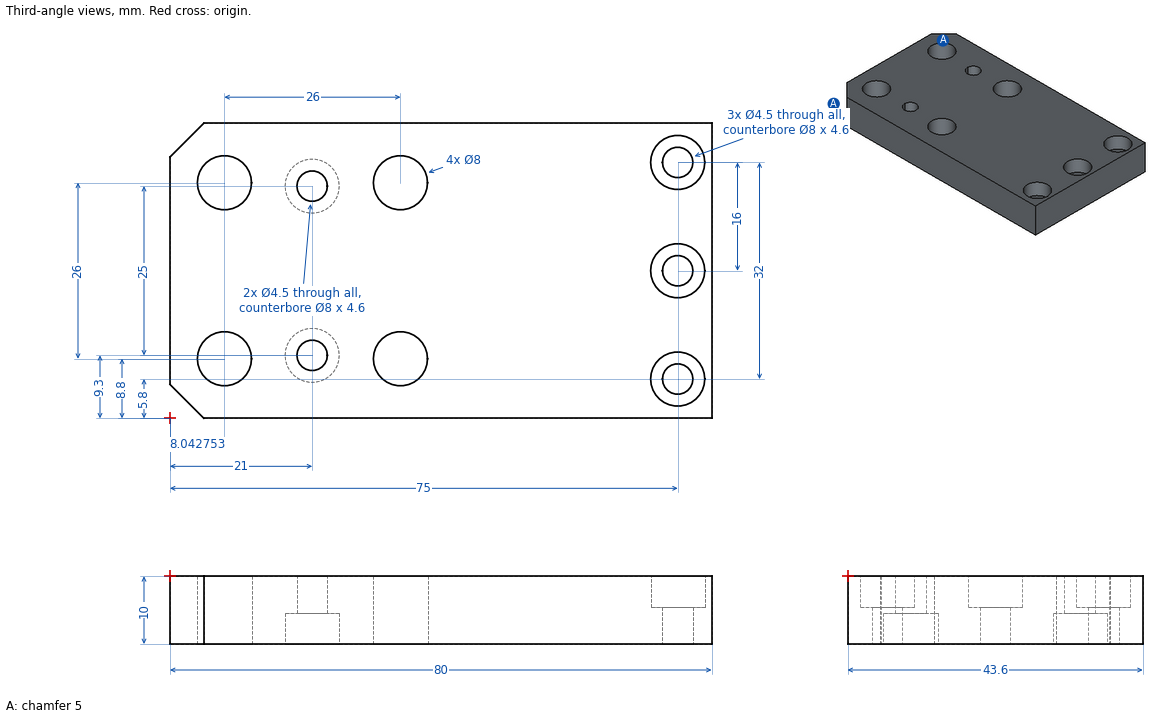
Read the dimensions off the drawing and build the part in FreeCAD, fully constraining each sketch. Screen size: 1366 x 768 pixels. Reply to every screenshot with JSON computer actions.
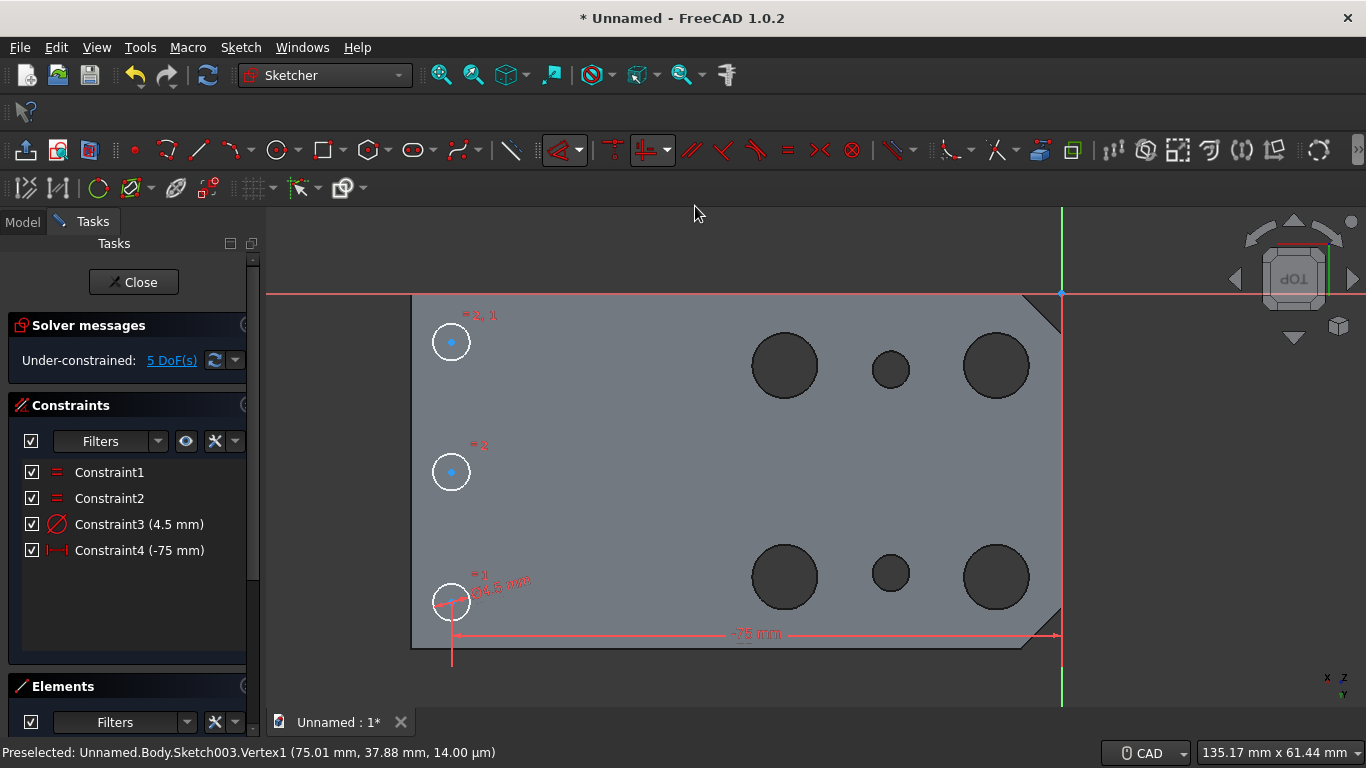
{"action": "left_click", "coordinate": [451, 342]}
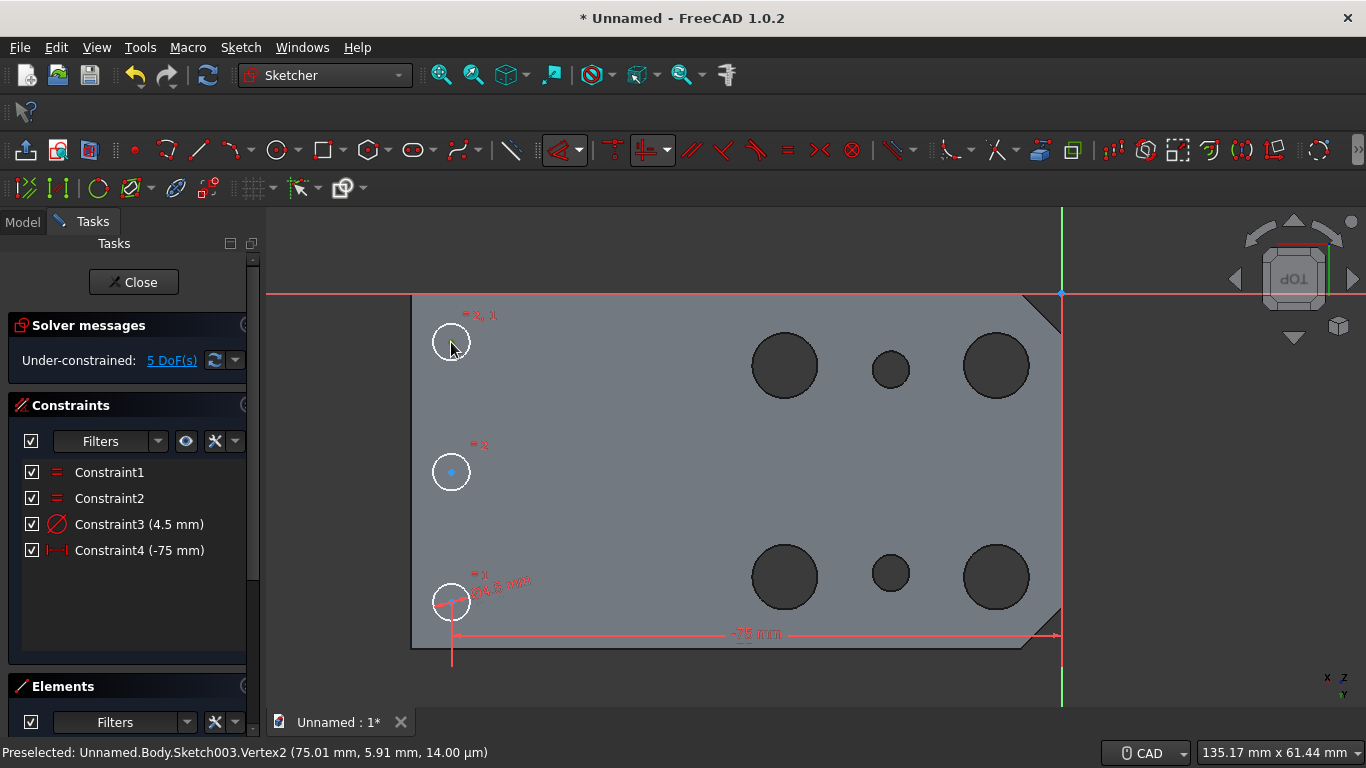
{"action": "left_click", "coordinate": [582, 150]}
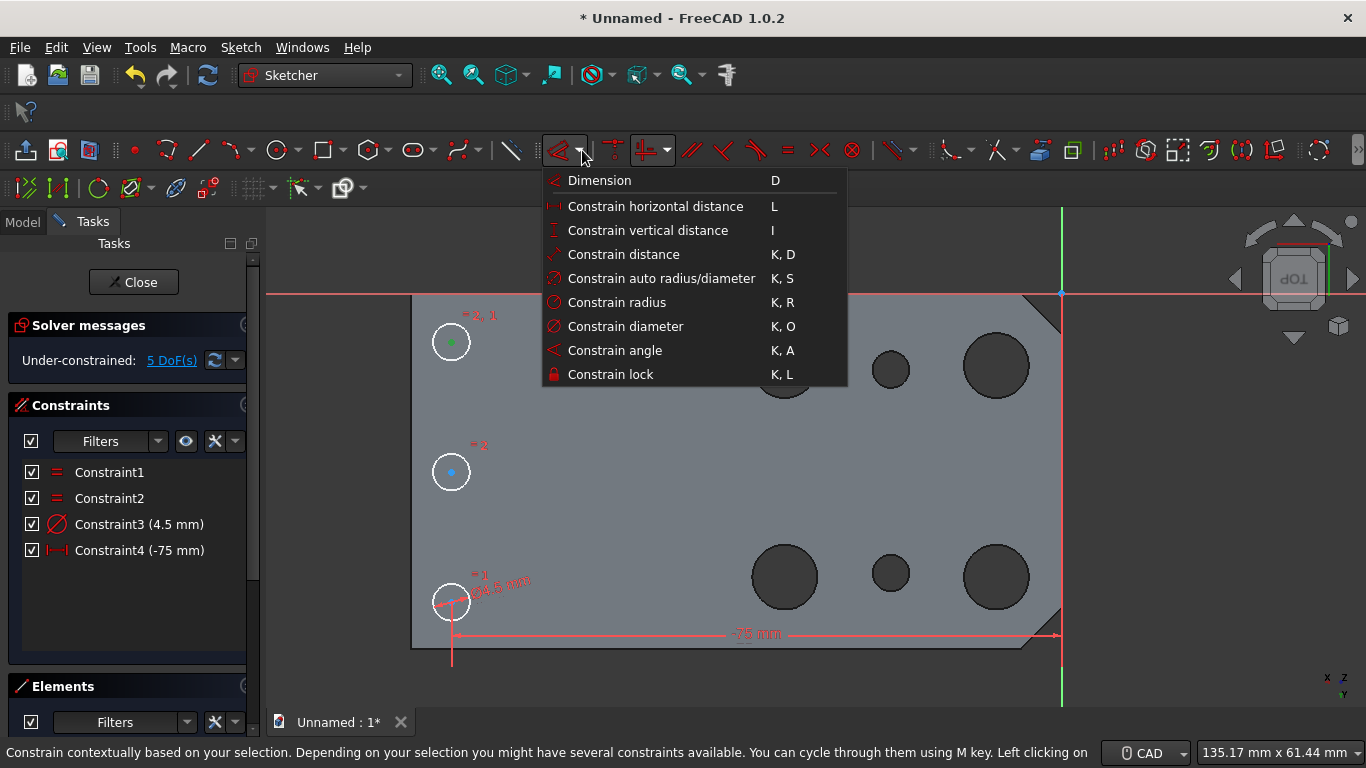
{"action": "left_click", "coordinate": [695, 206]}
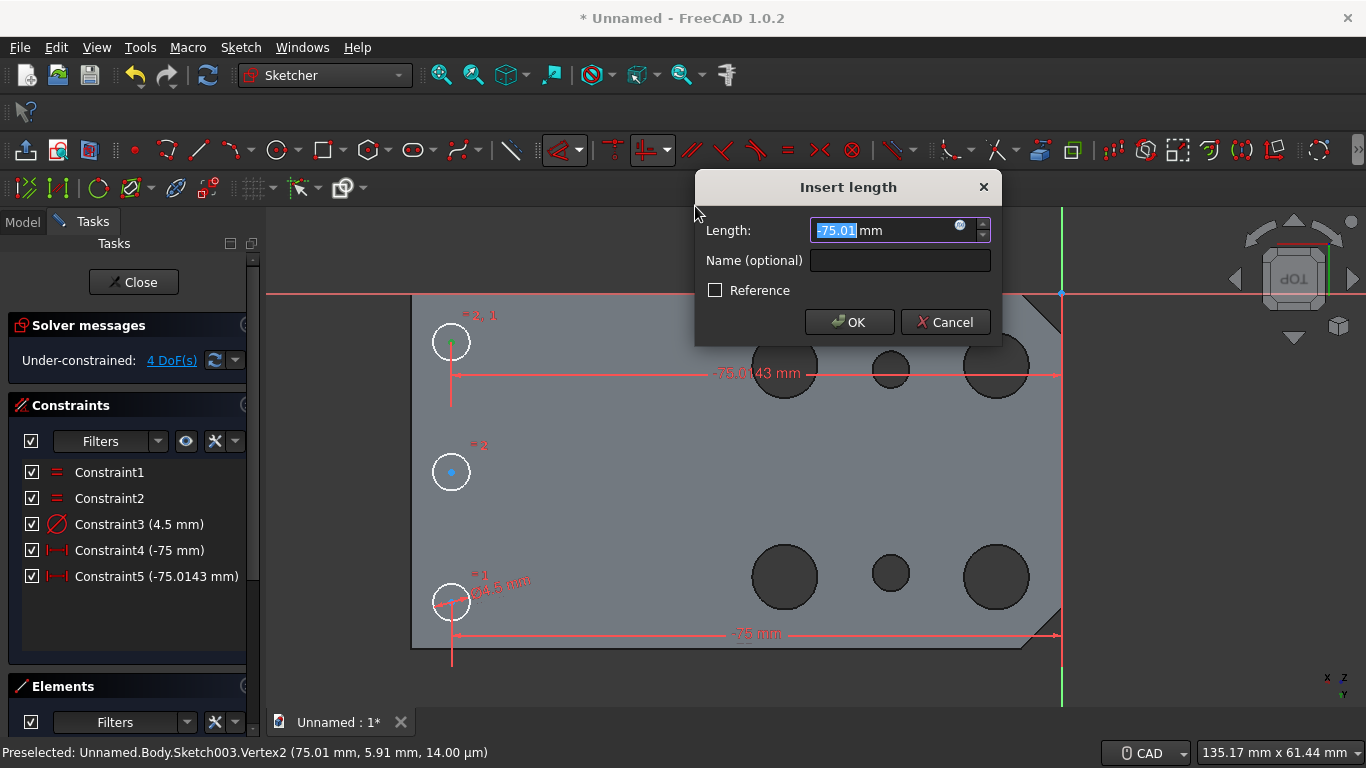
{"action": "type", "text": "-75"}
{"action": "key", "text": "Return"}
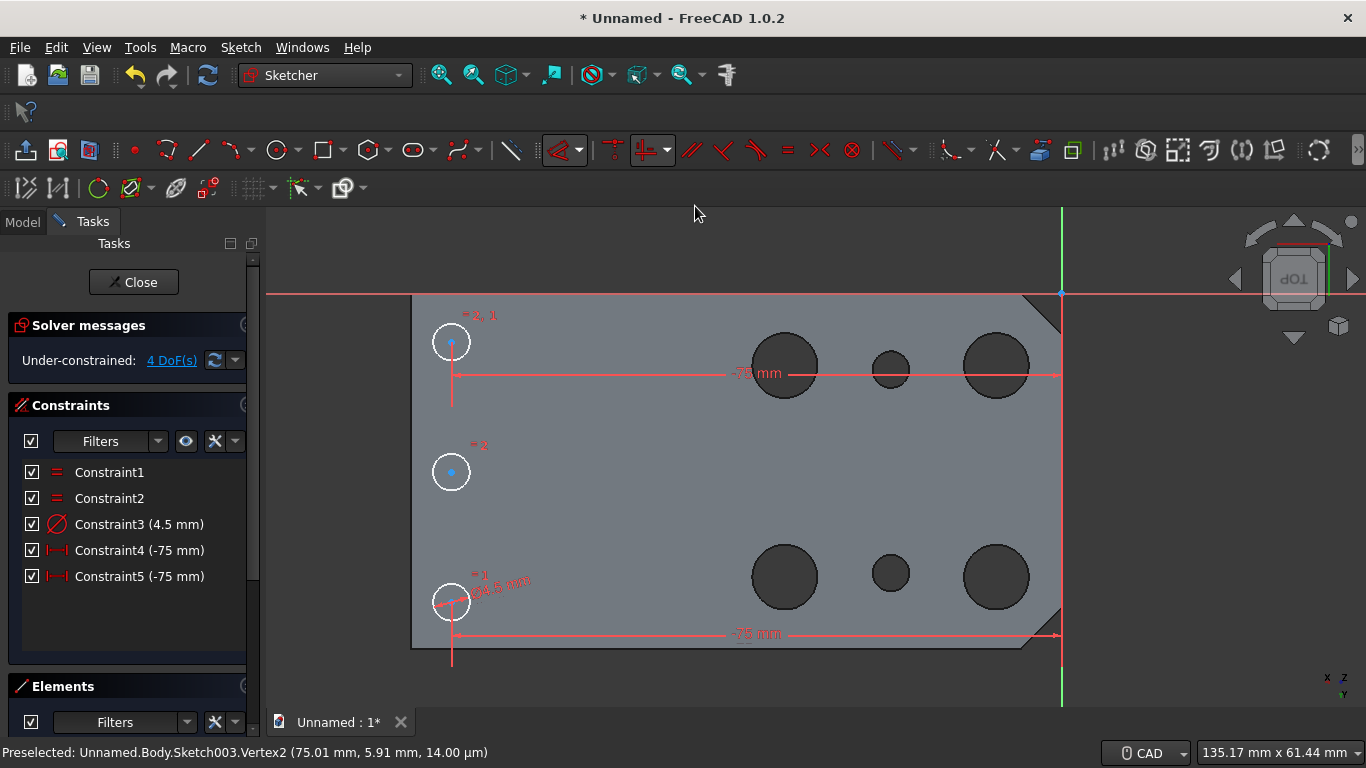
{"action": "left_click", "coordinate": [451, 472]}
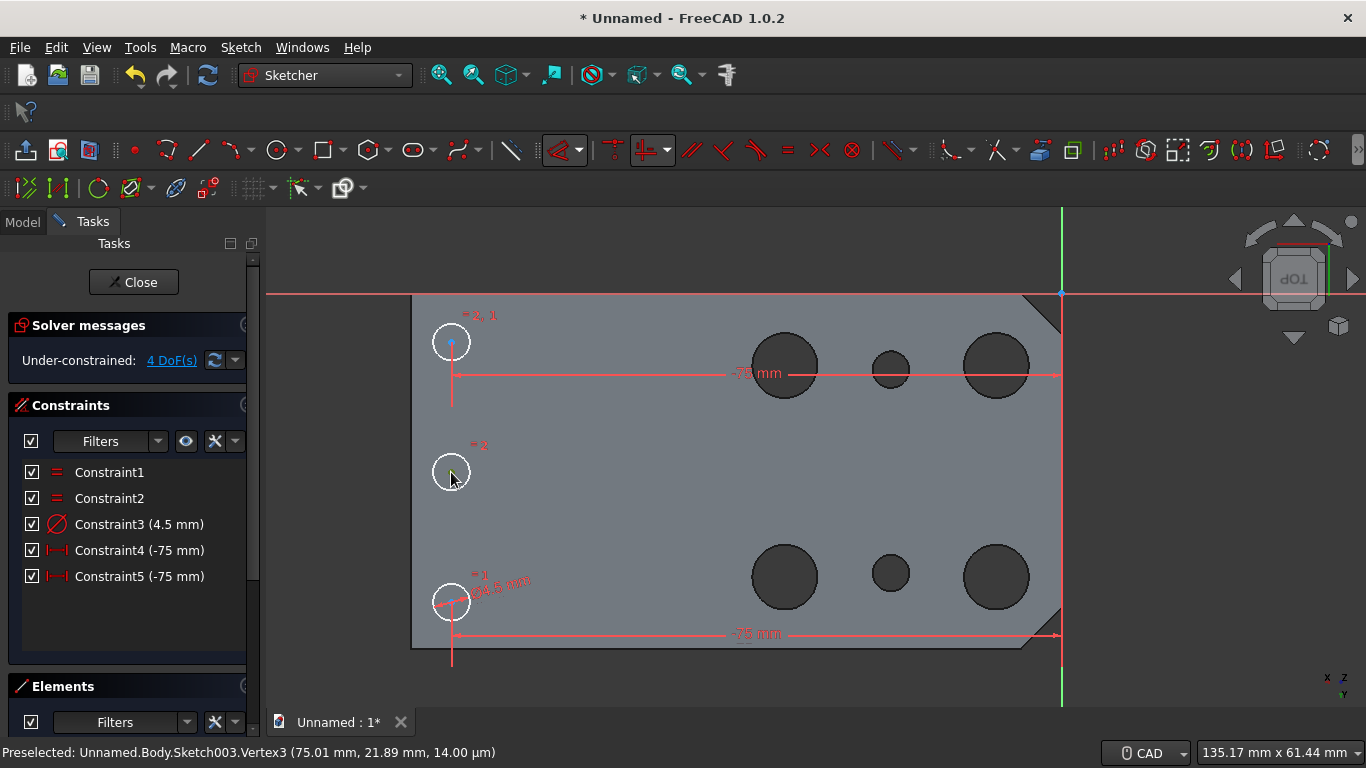
{"action": "left_click", "coordinate": [582, 150]}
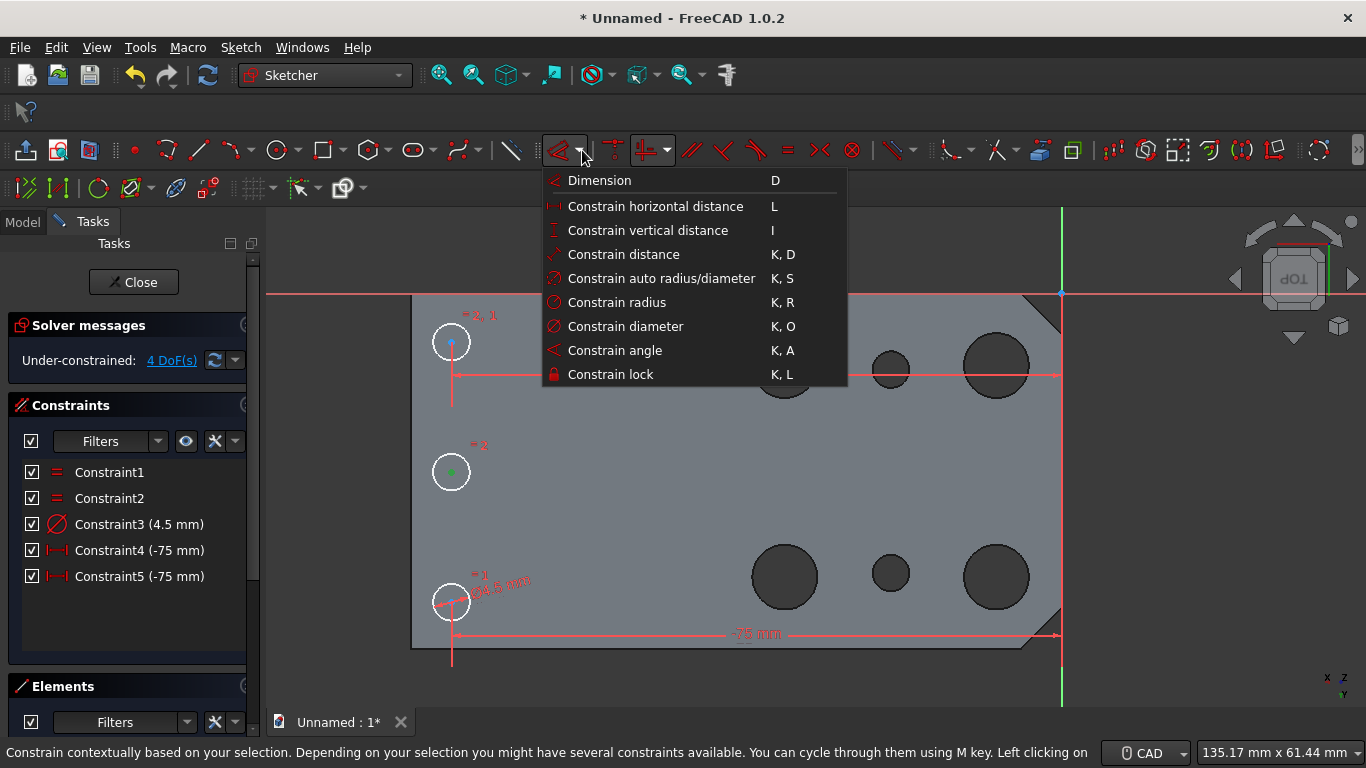
{"action": "left_click", "coordinate": [695, 206]}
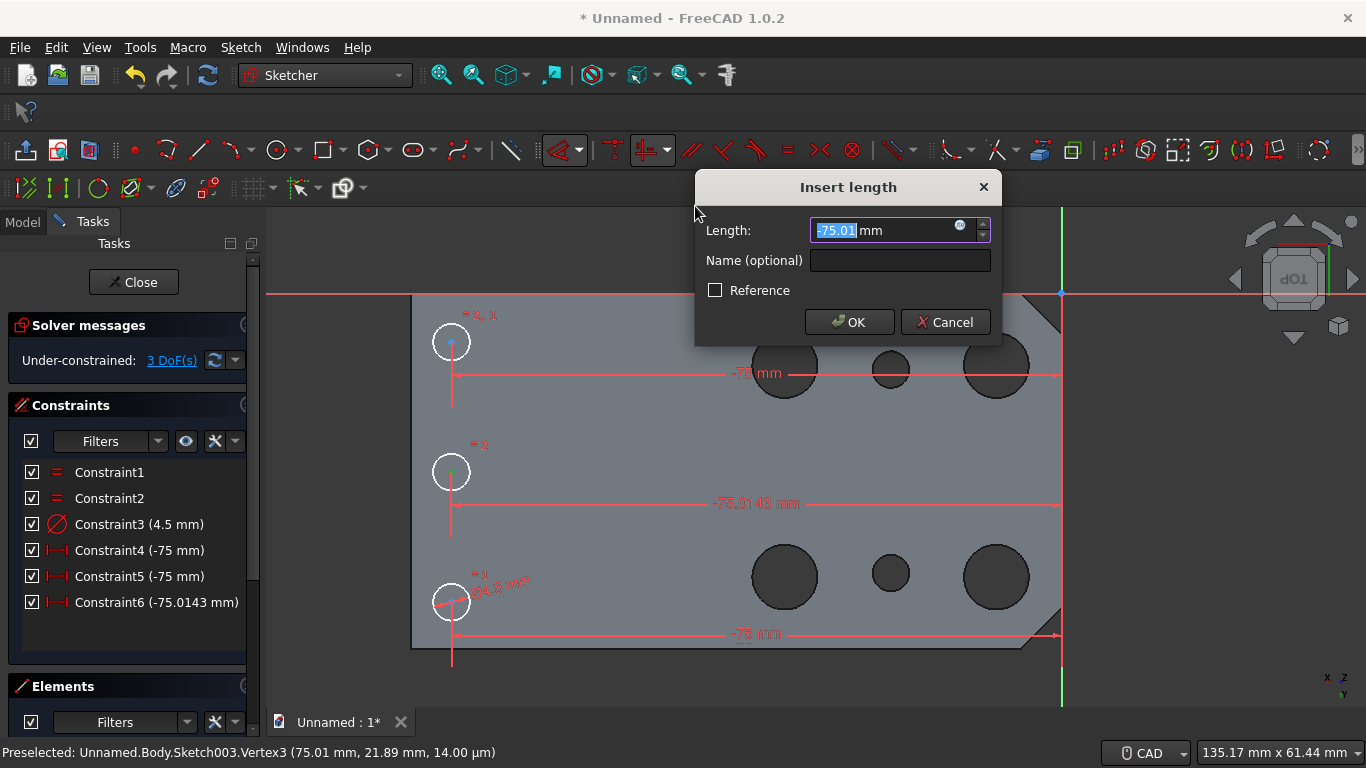
{"action": "type", "text": "-75"}
{"action": "key", "text": "Return"}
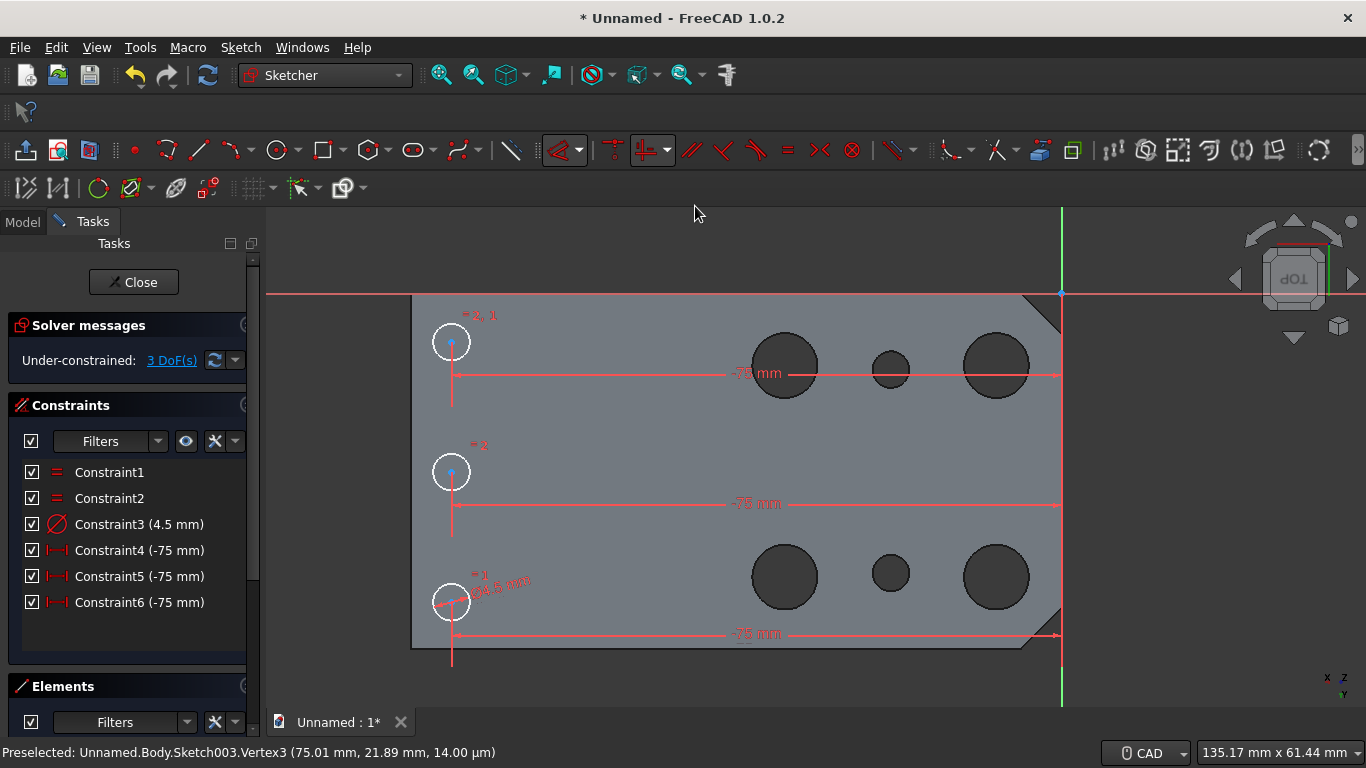
{"action": "left_click", "coordinate": [452, 342]}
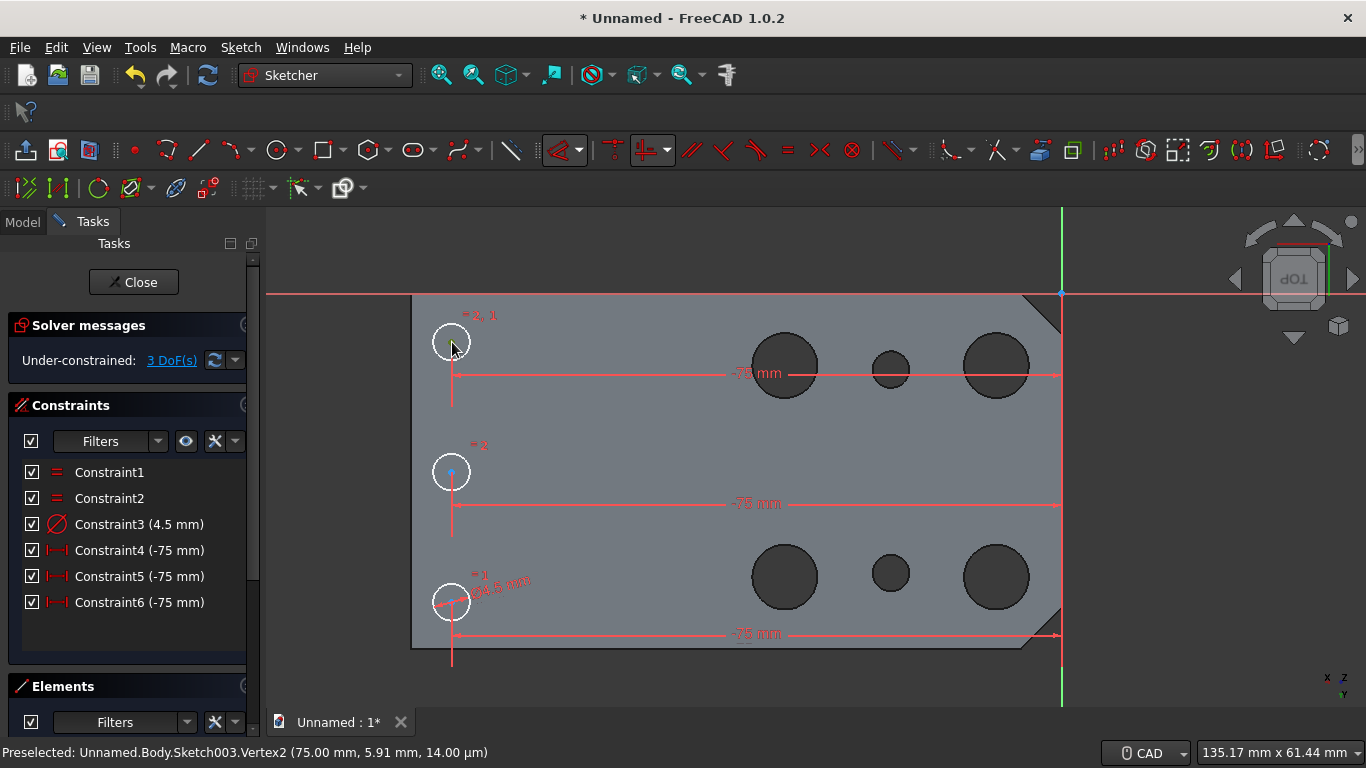
{"action": "key", "text": "i"}